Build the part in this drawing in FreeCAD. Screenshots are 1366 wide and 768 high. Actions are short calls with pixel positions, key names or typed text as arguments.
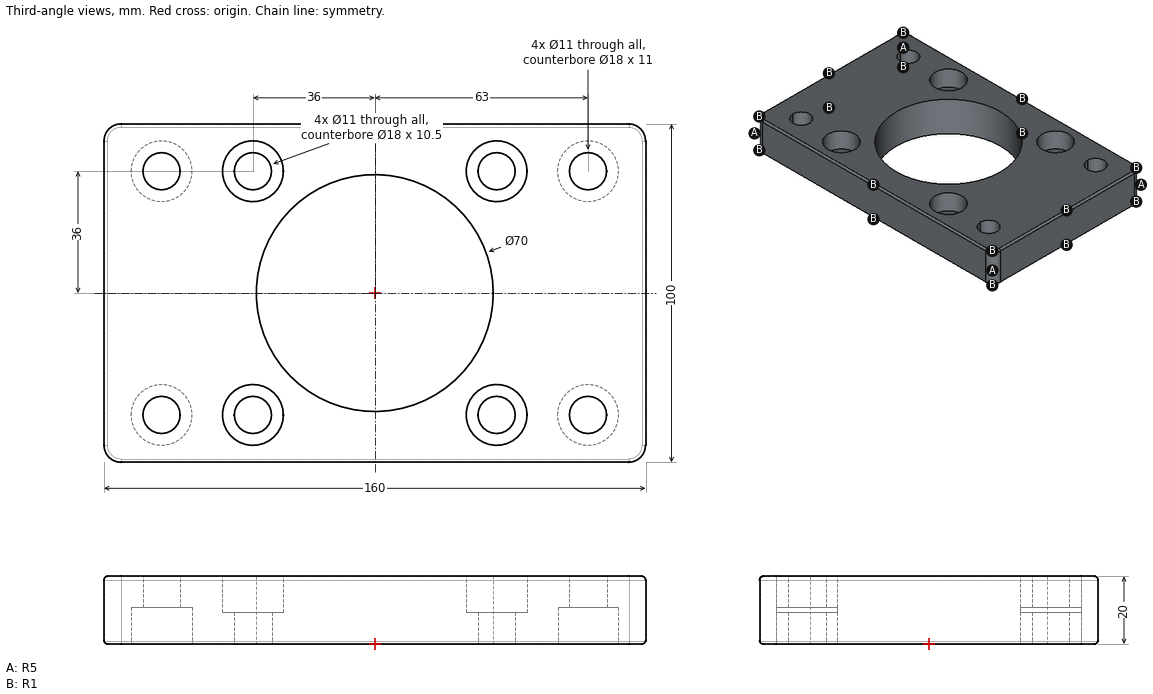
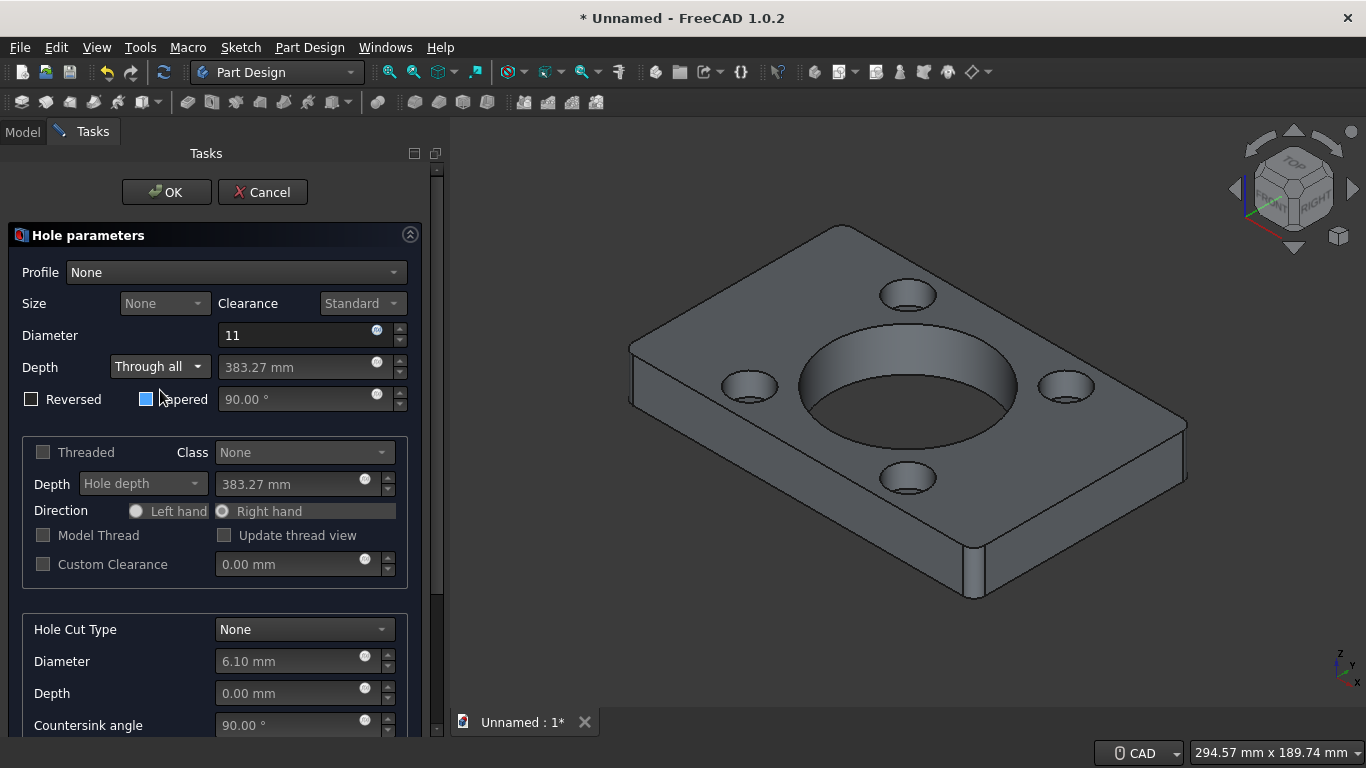
click(30, 399)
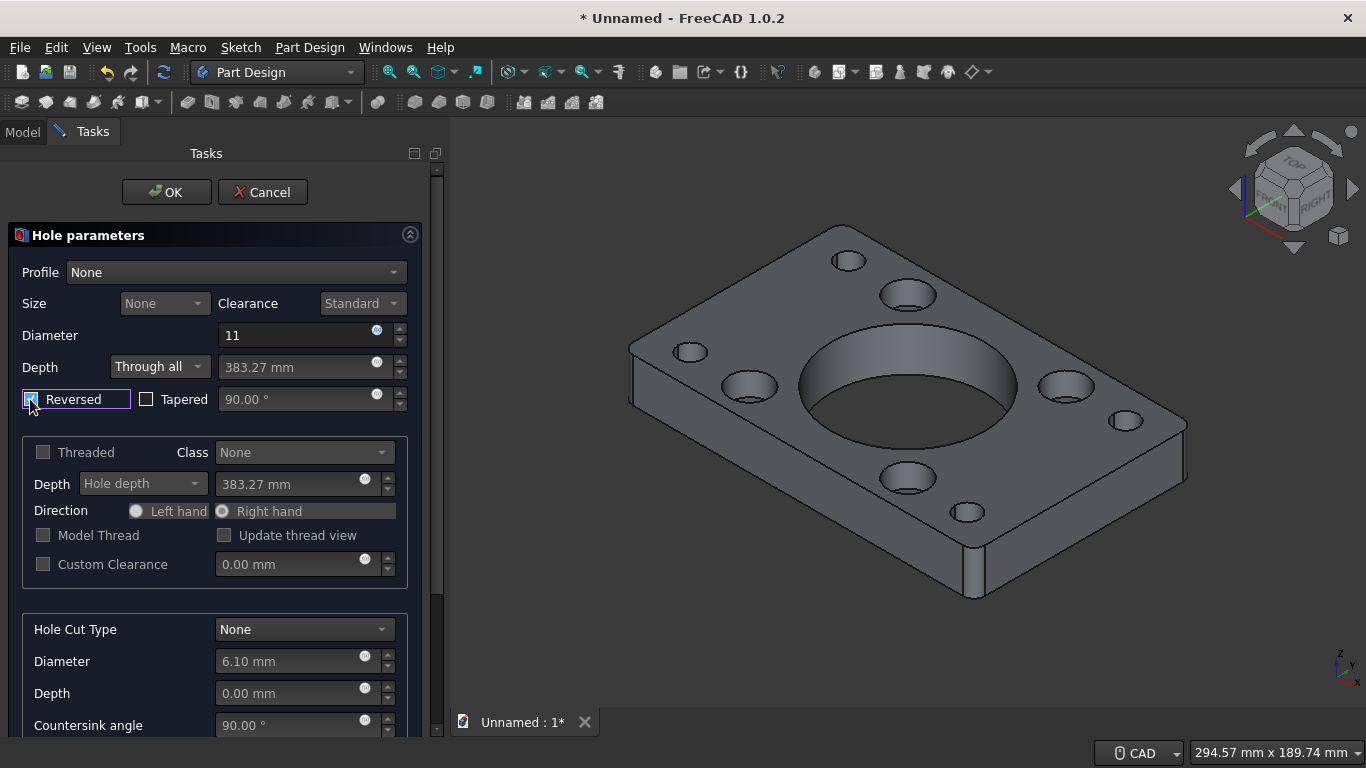
click(306, 630)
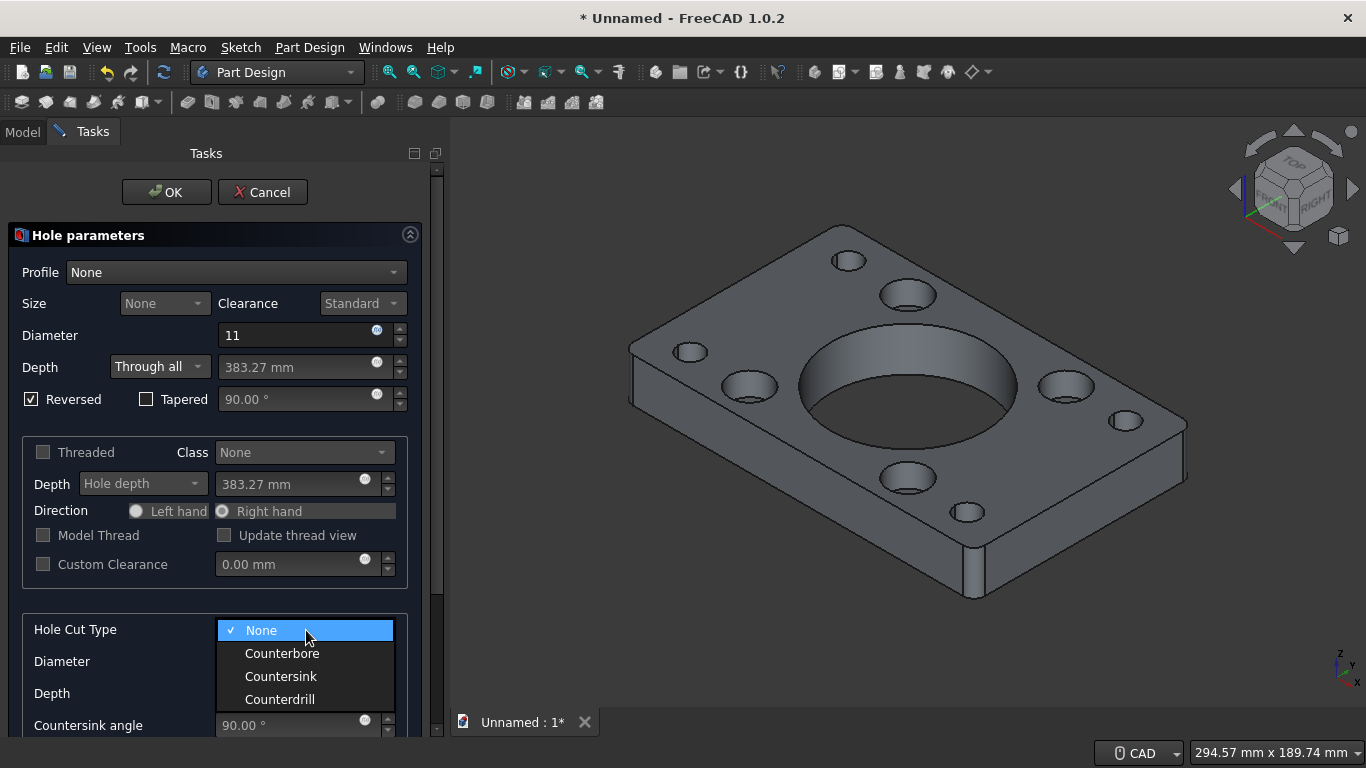
click(304, 654)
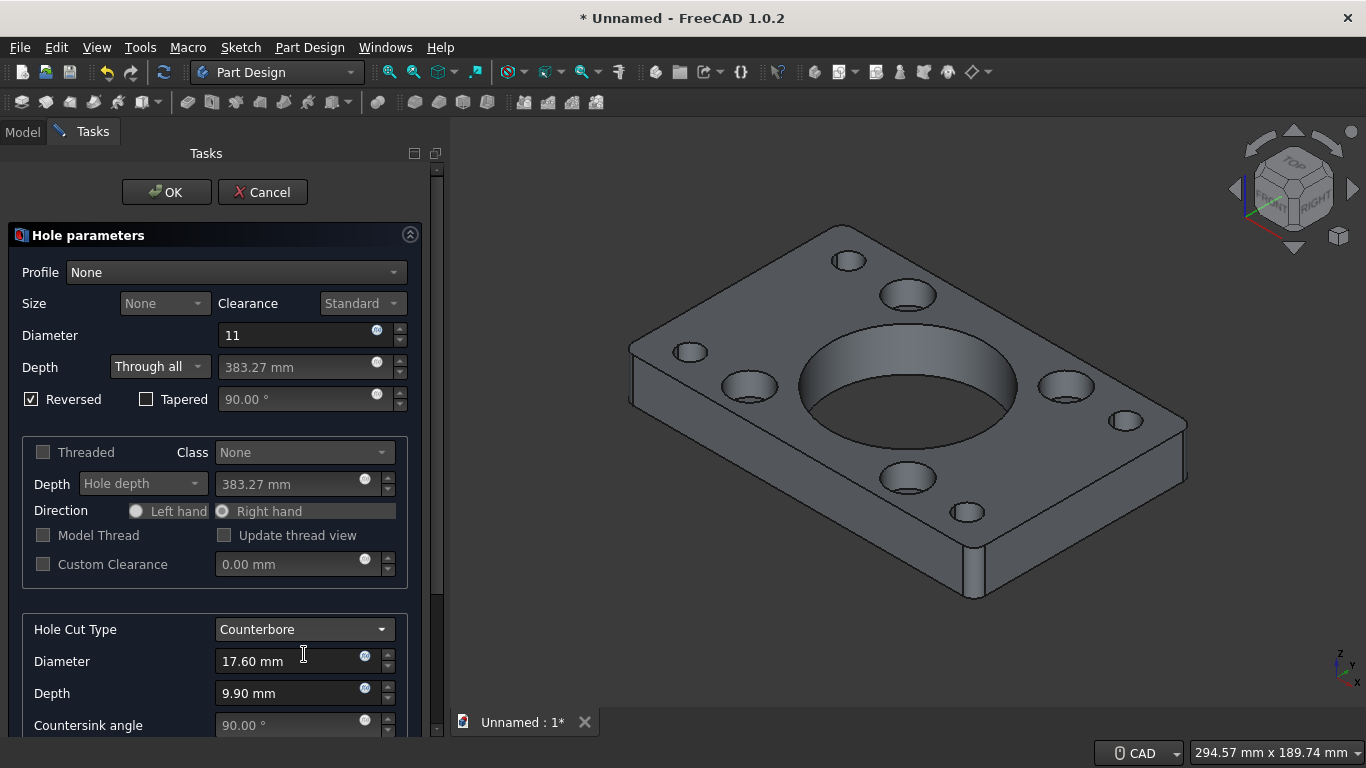
triple_click(298, 661)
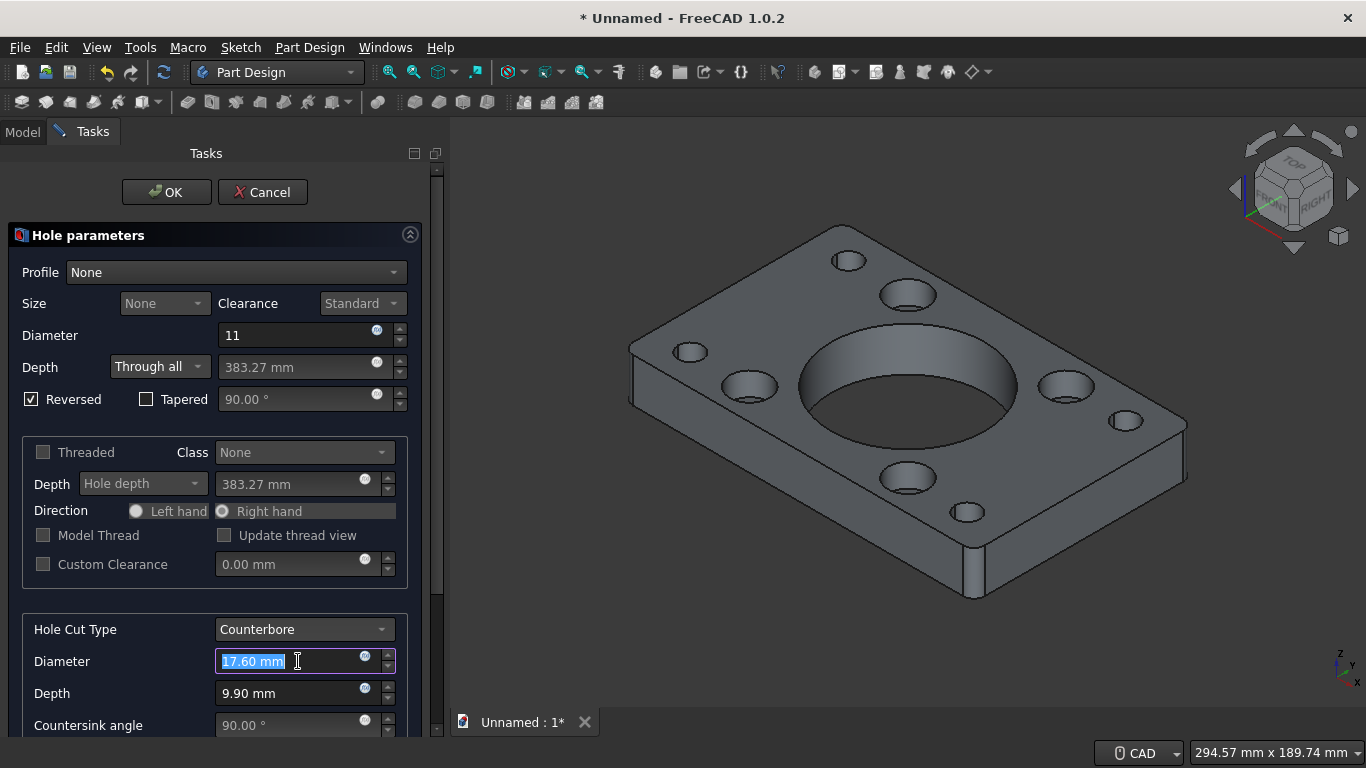
text(18)
key(Tab)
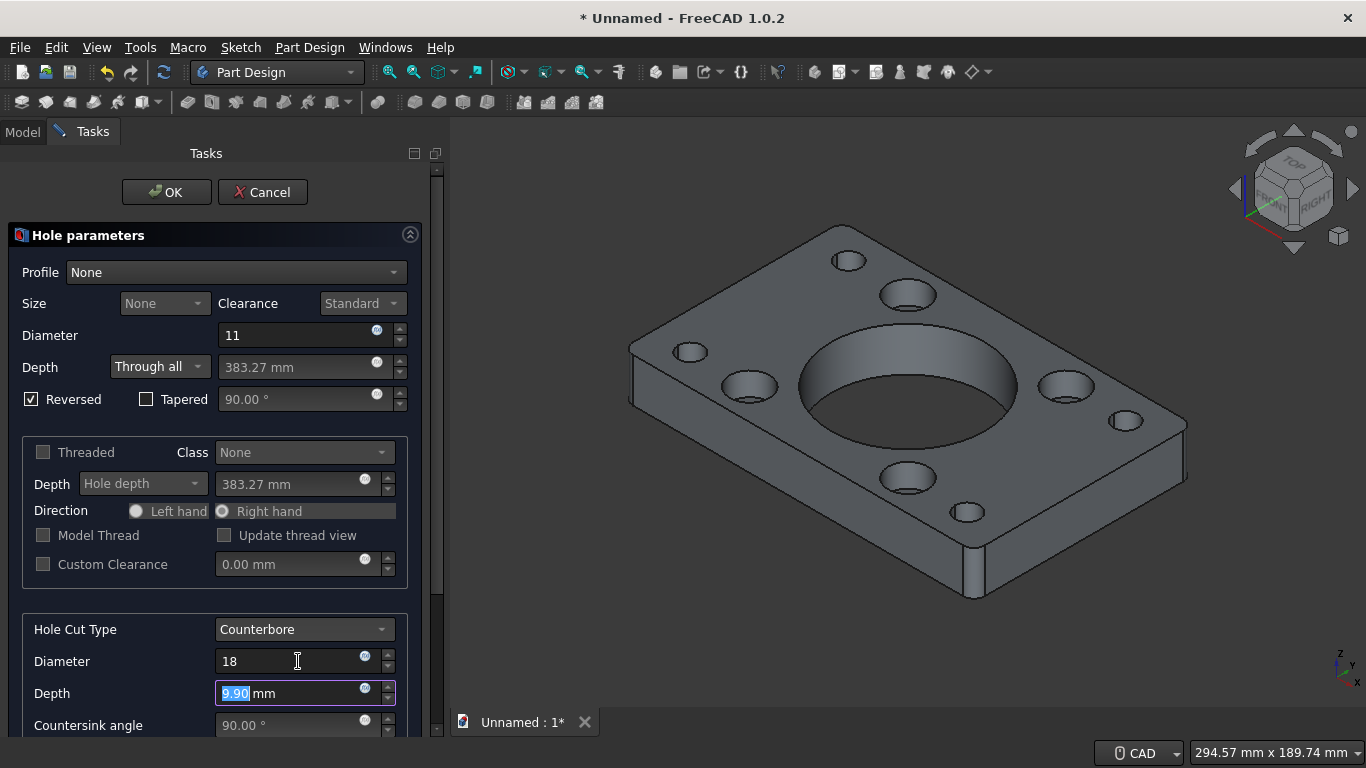
text(11)
key(Tab)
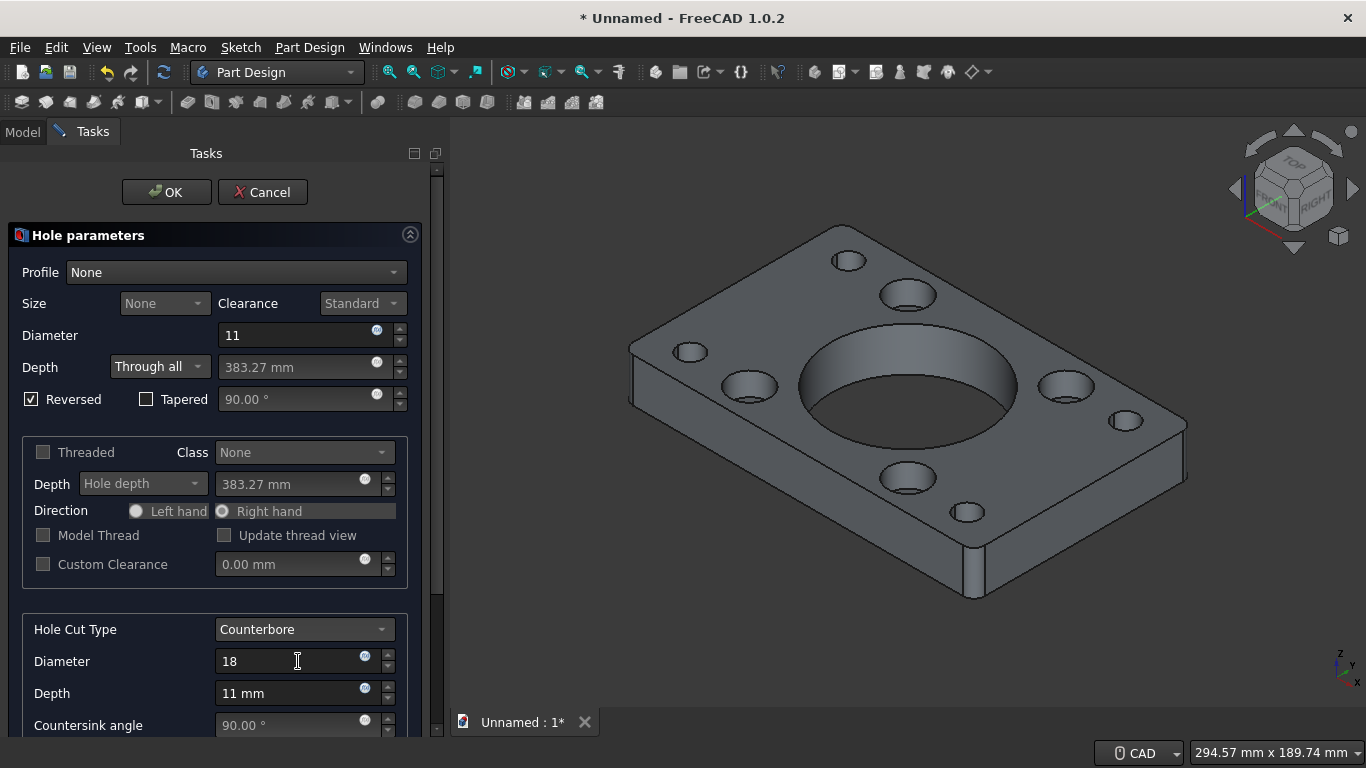
click(167, 192)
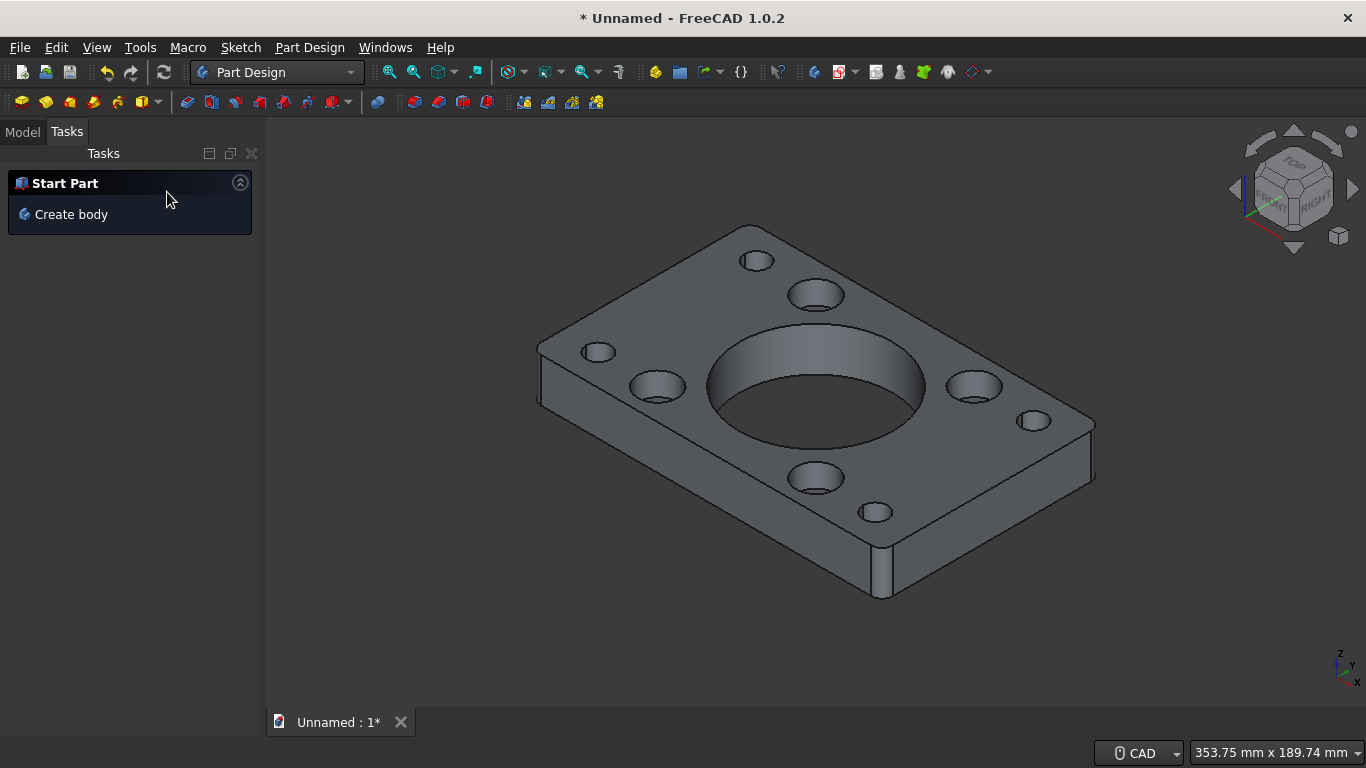
click(992, 487)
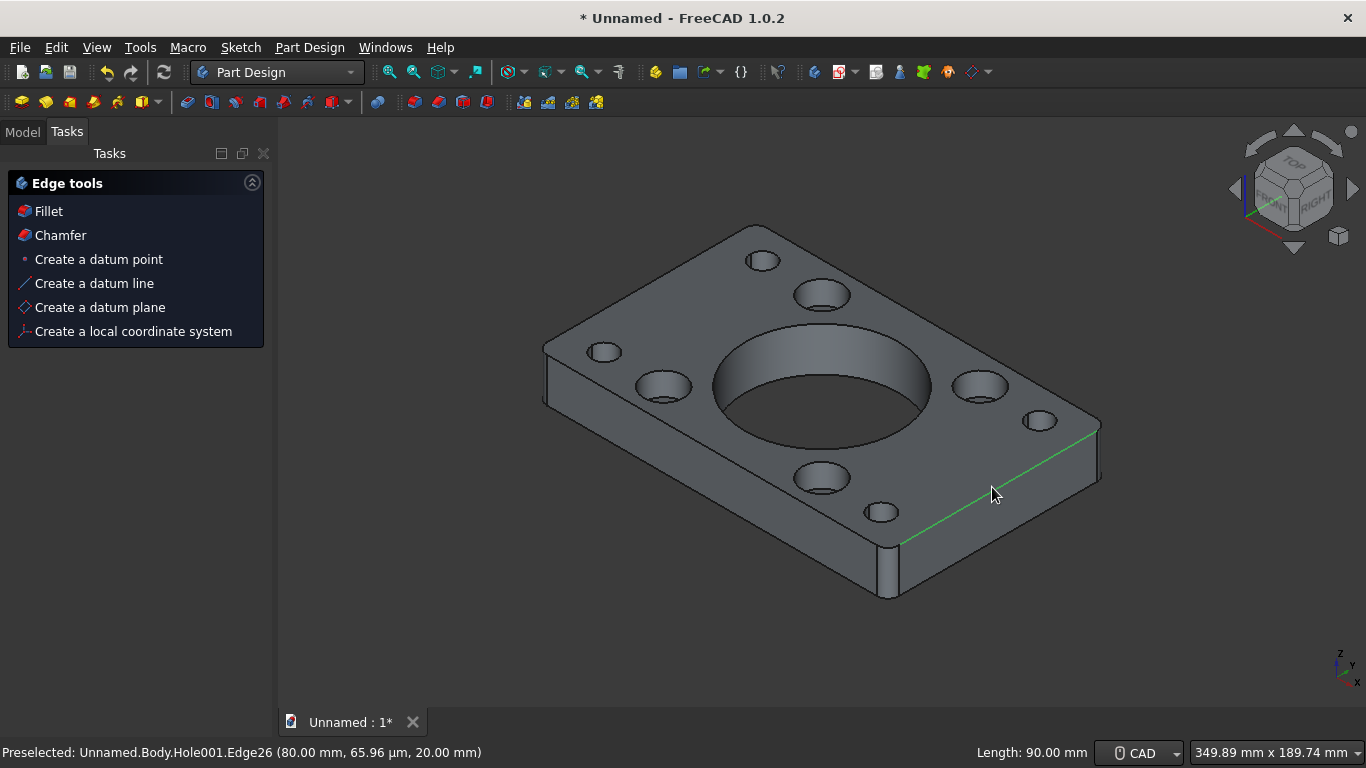
click(881, 597, ctrl)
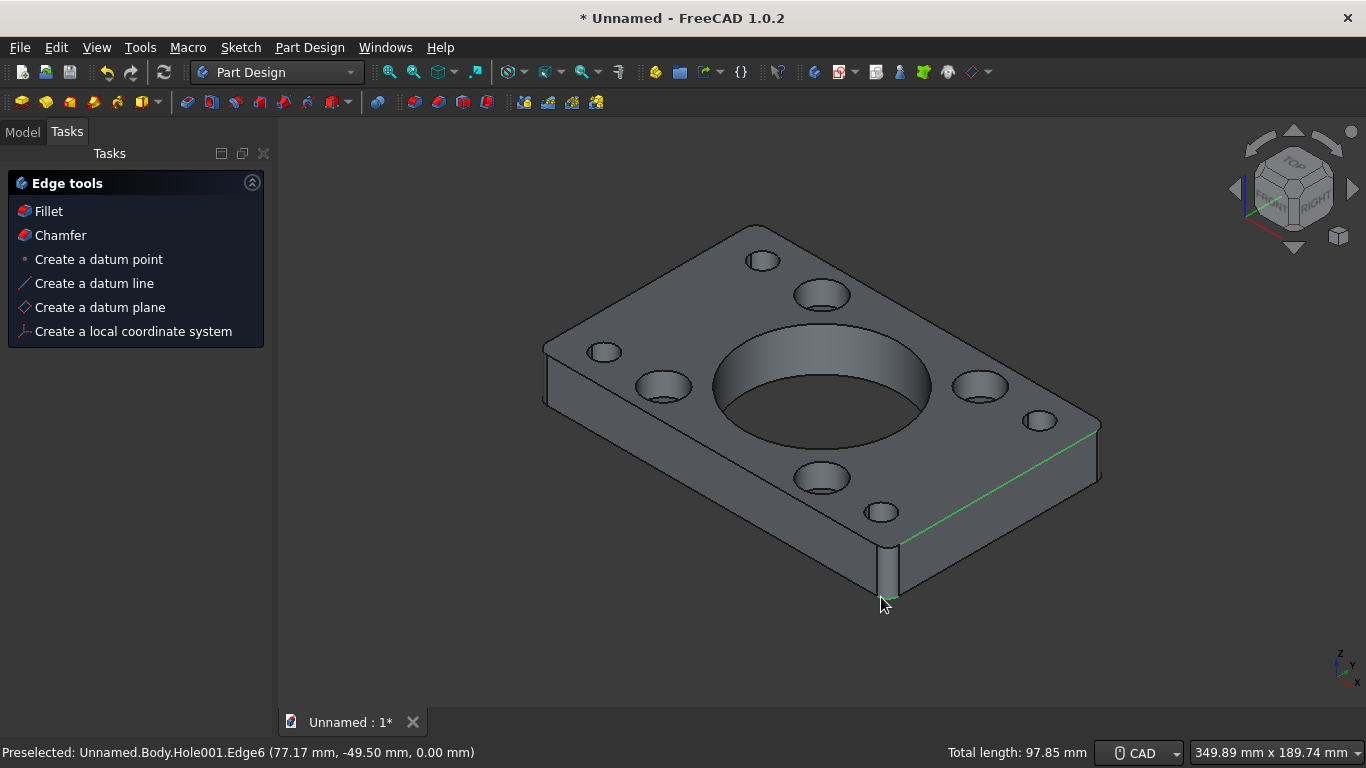
click(712, 449, ctrl)